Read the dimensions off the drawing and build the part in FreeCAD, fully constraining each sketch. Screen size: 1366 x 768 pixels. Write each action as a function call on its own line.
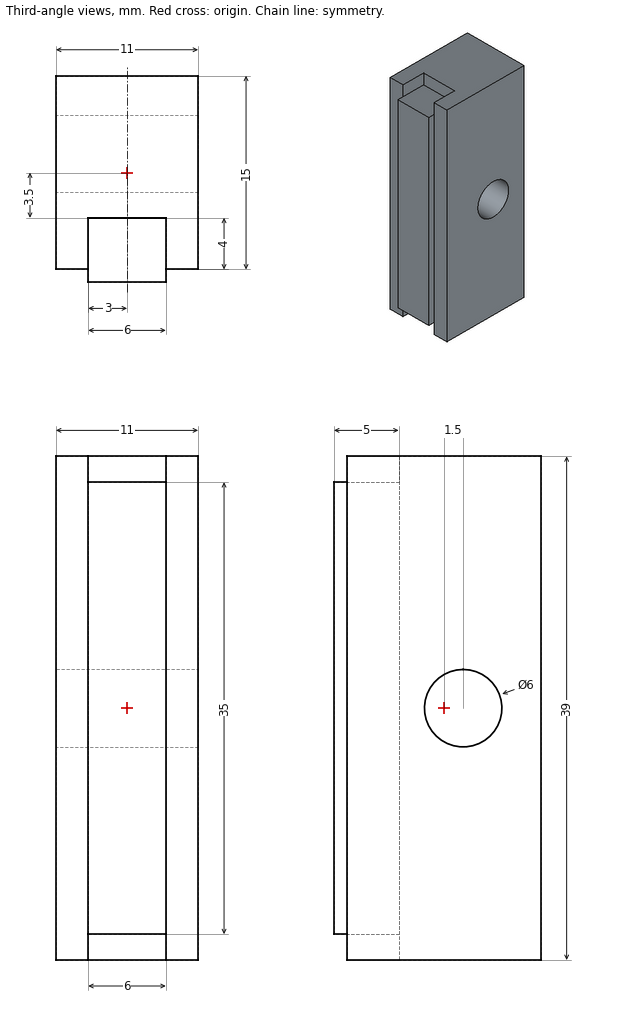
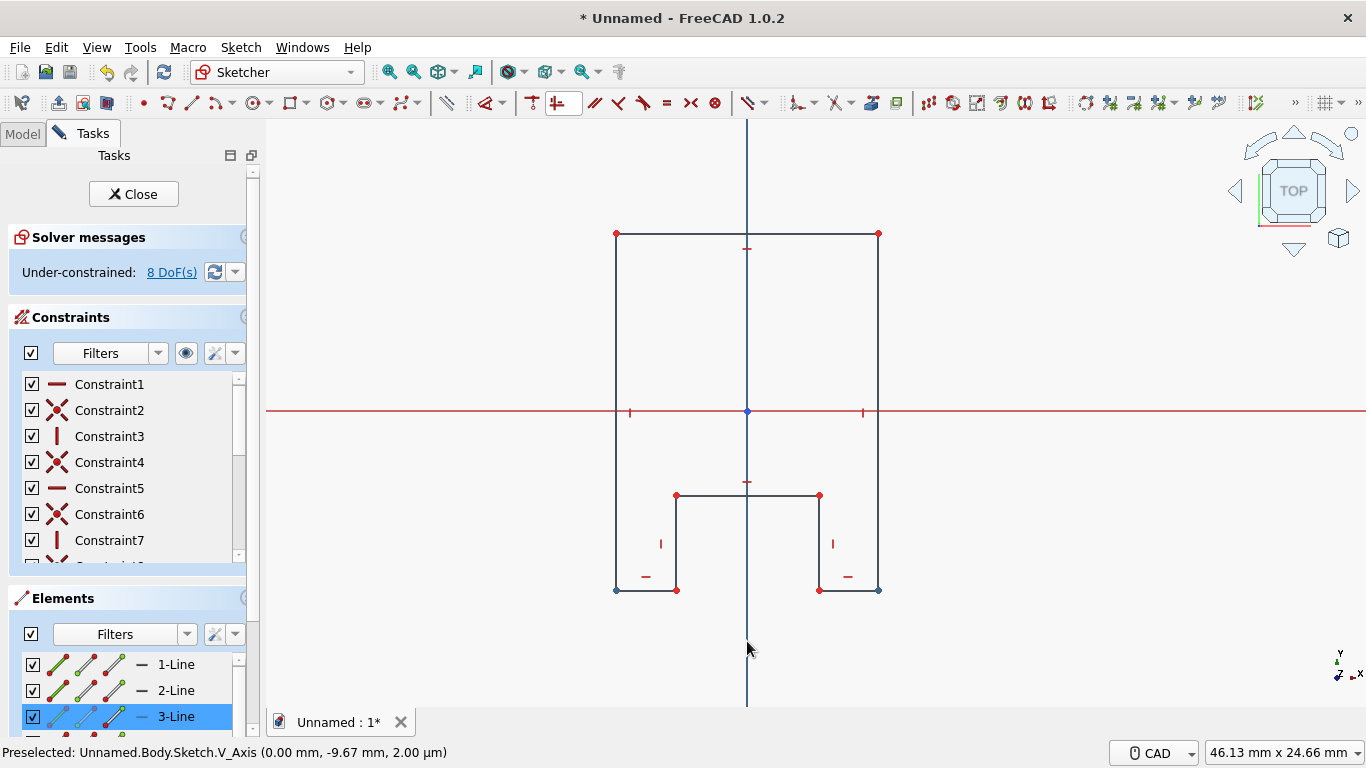
click(692, 104)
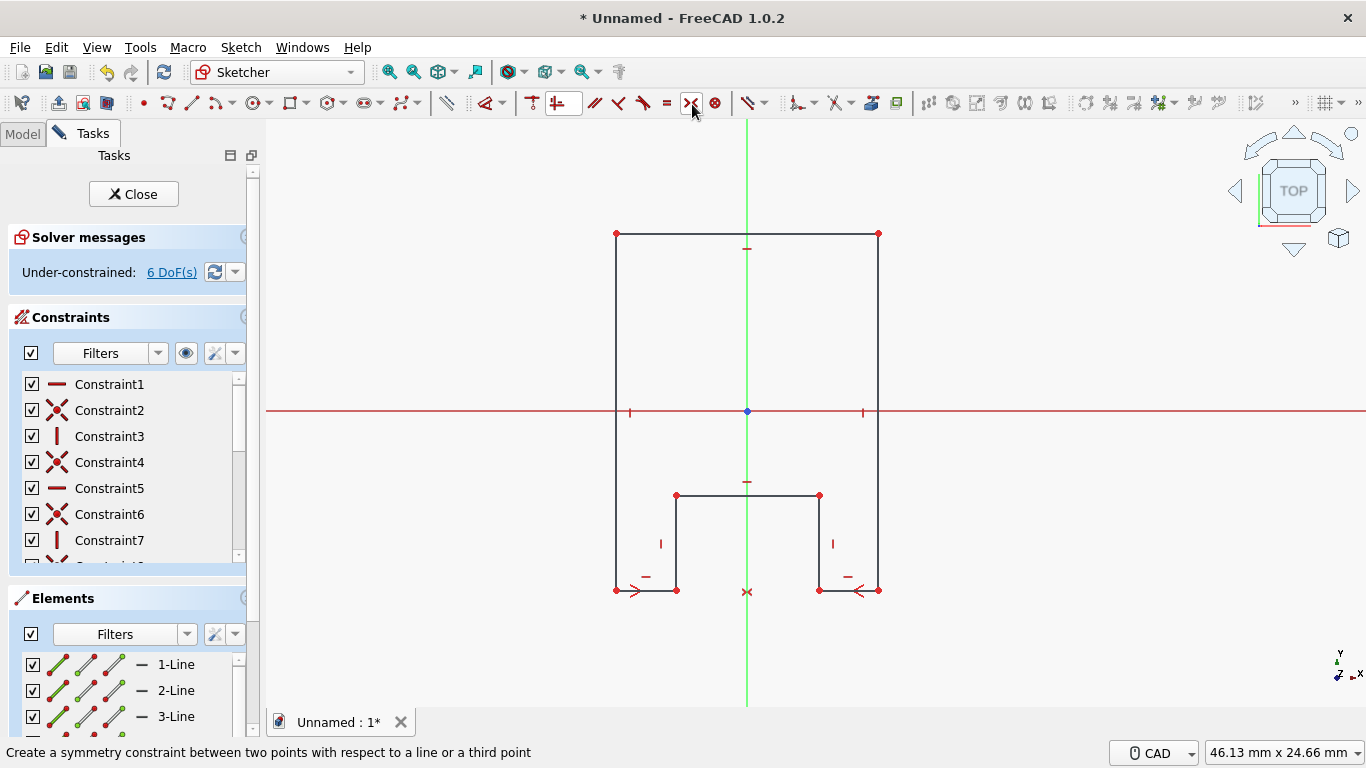
click(486, 104)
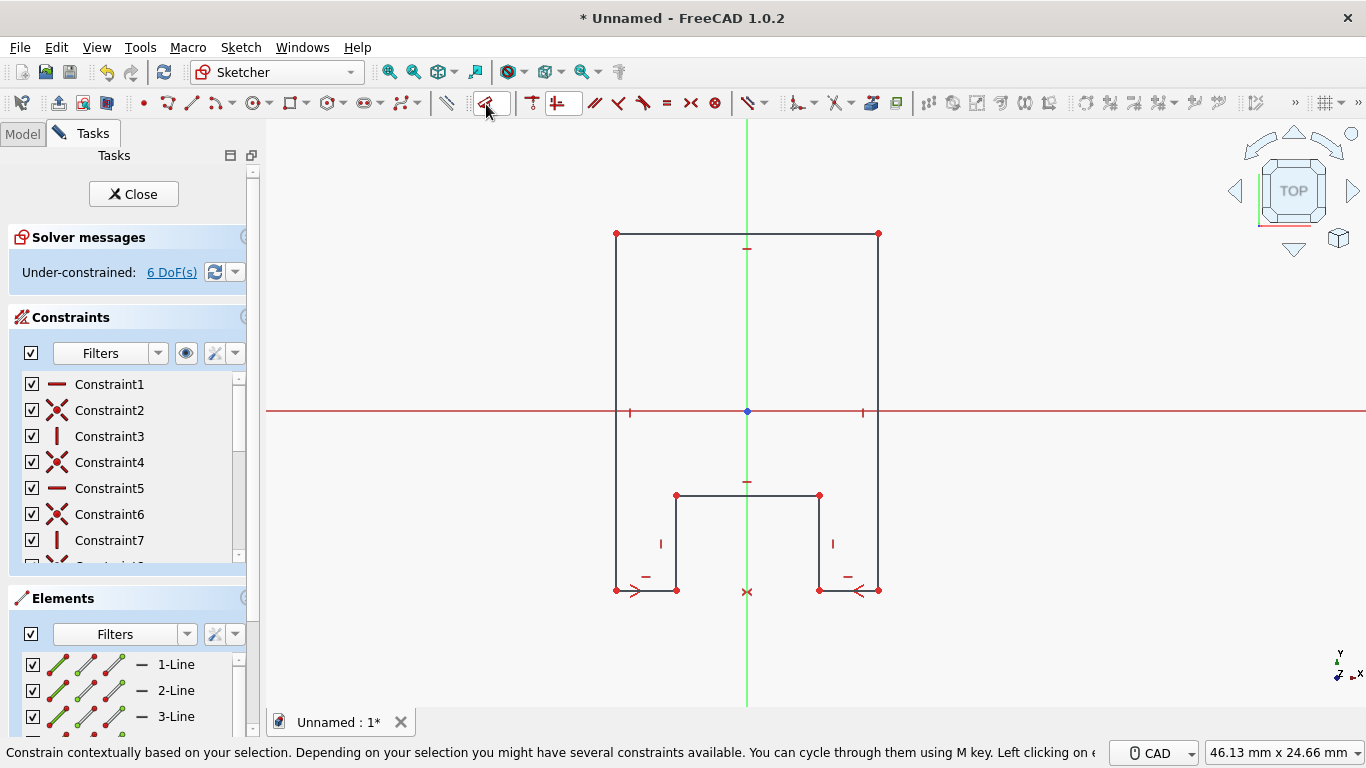
click(719, 496)
click(715, 530)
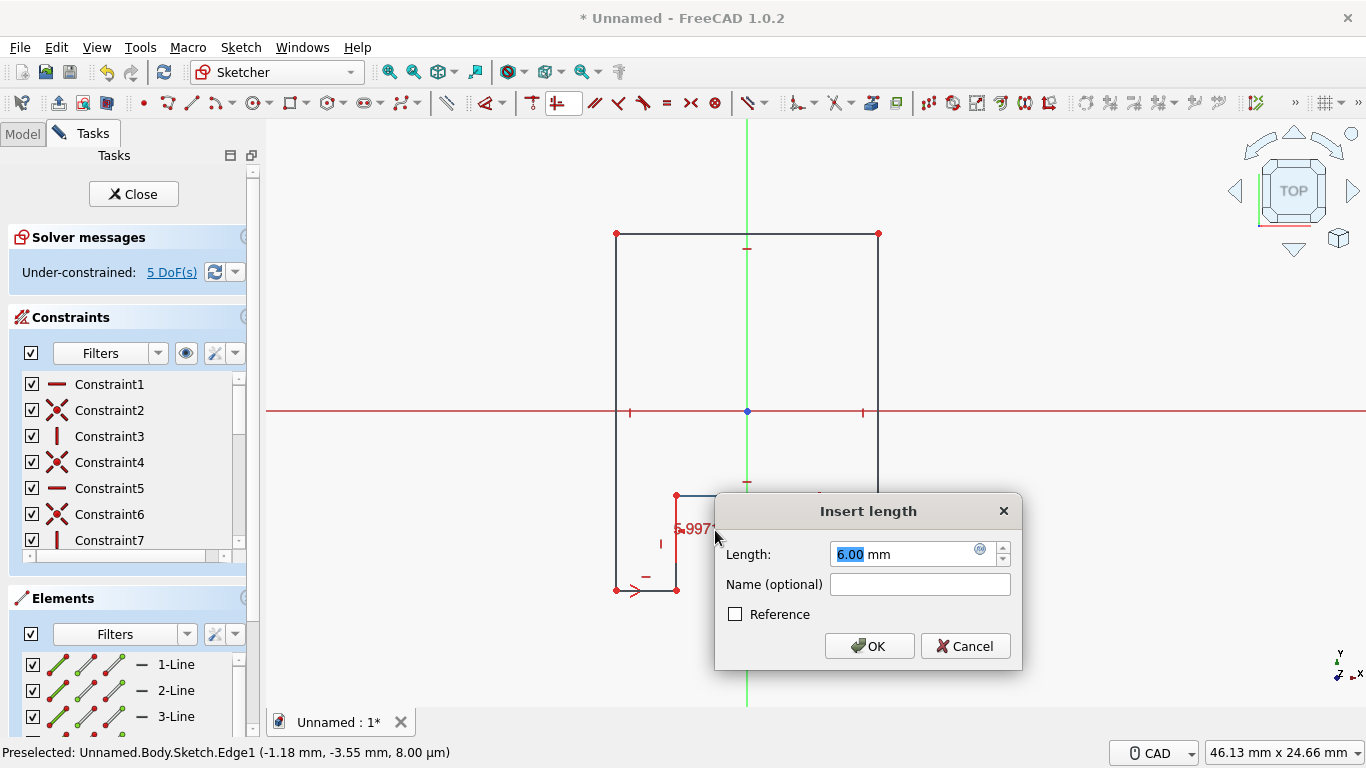
text(6)
key(Return)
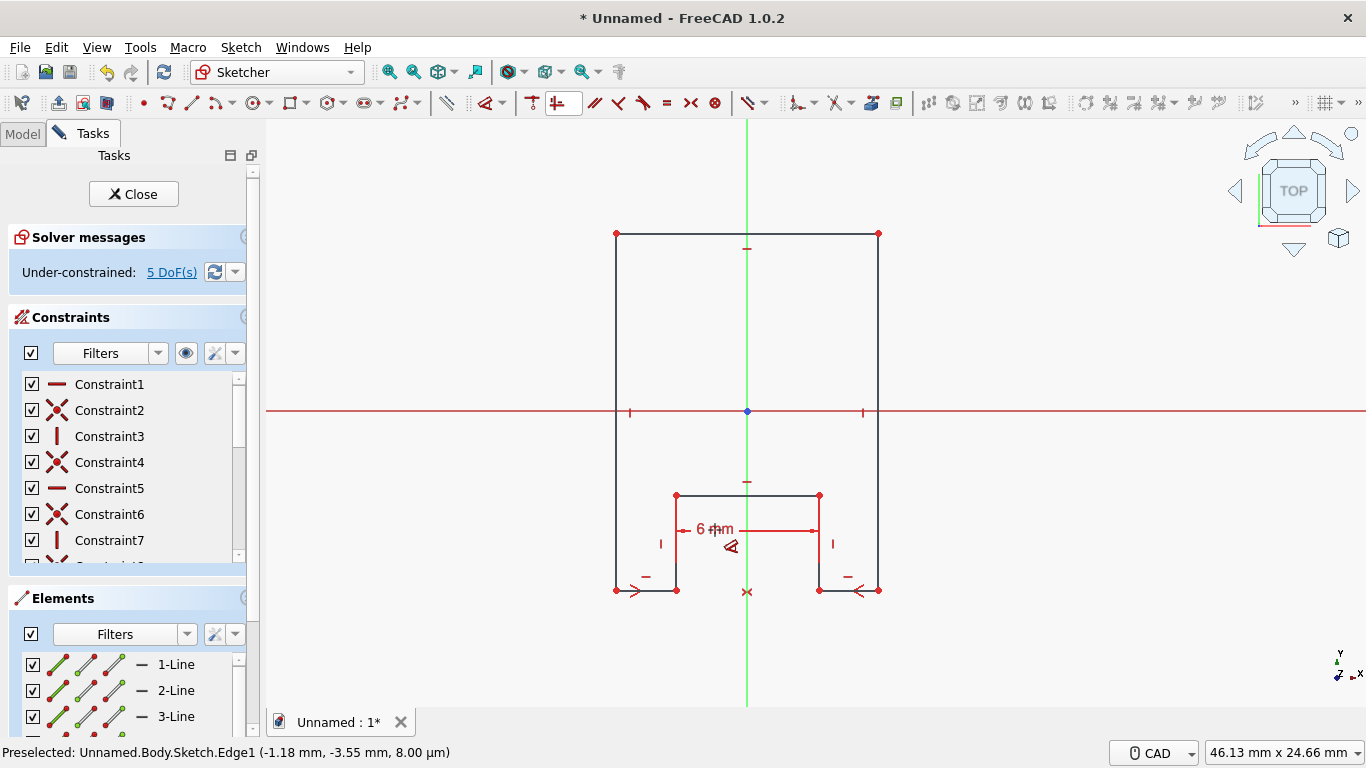
click(819, 524)
click(853, 543)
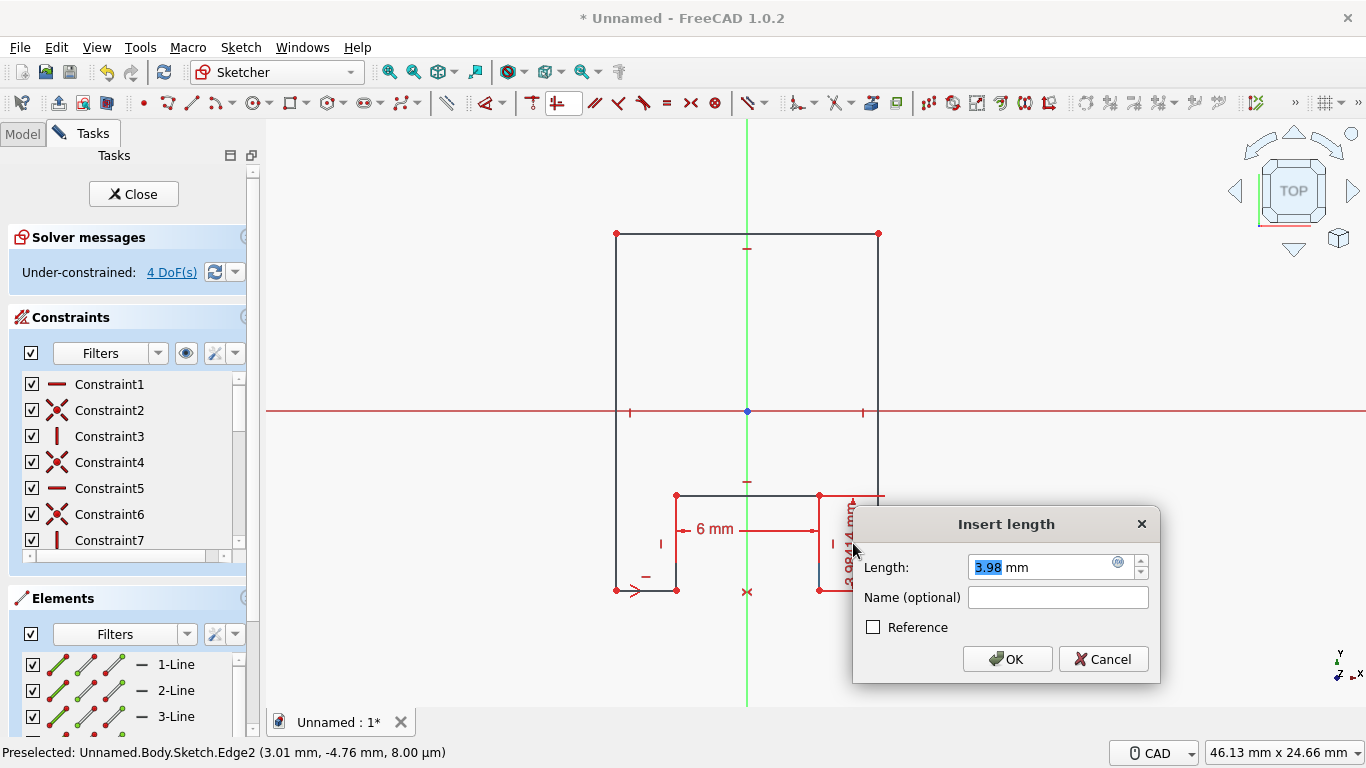
text(4)
key(Return)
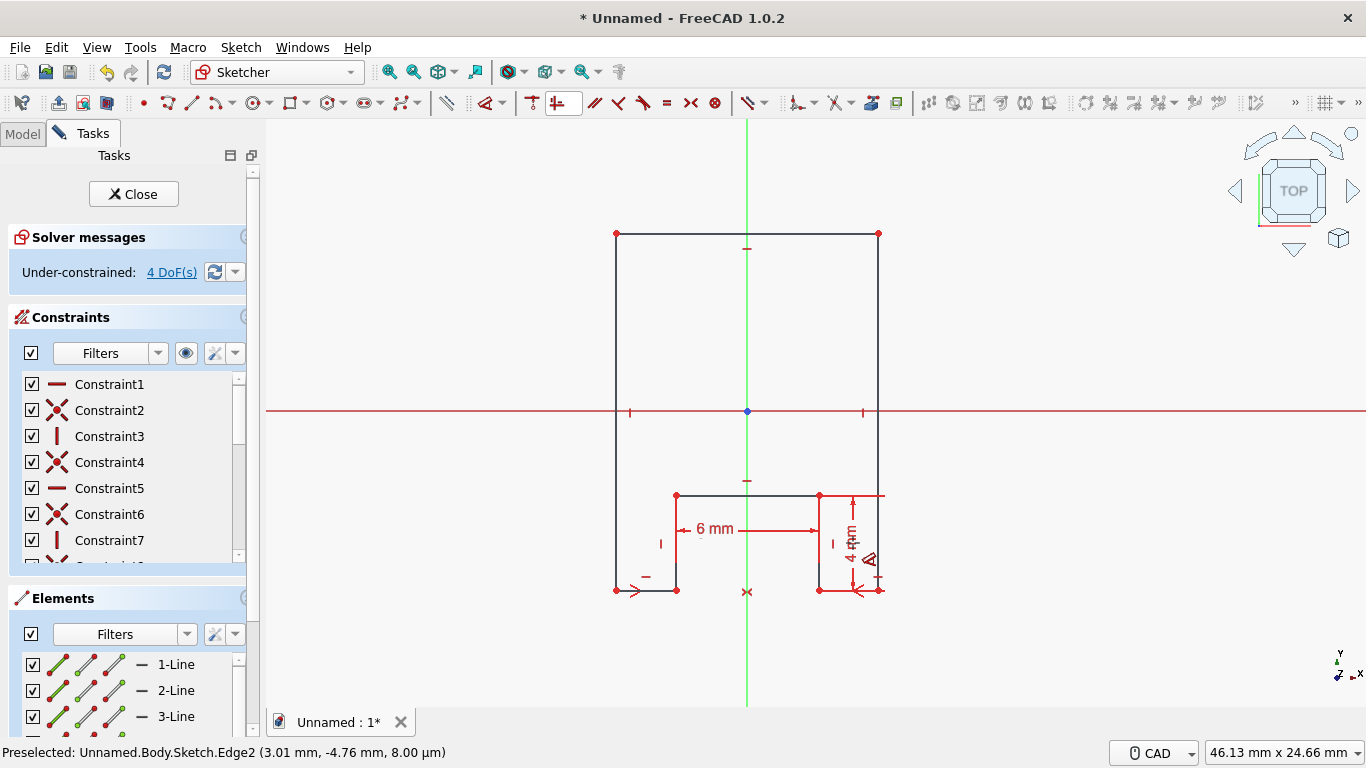
click(878, 484)
click(912, 330)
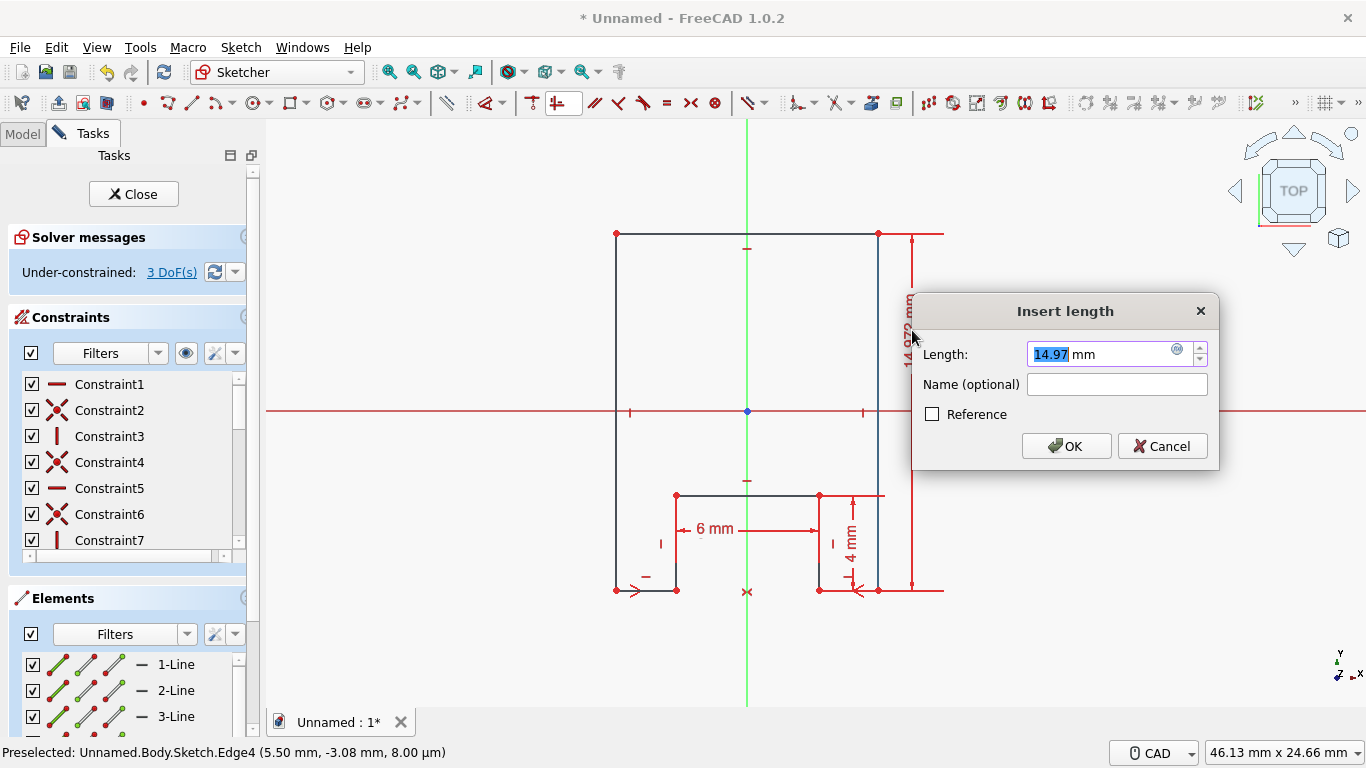
text(15)
key(Return)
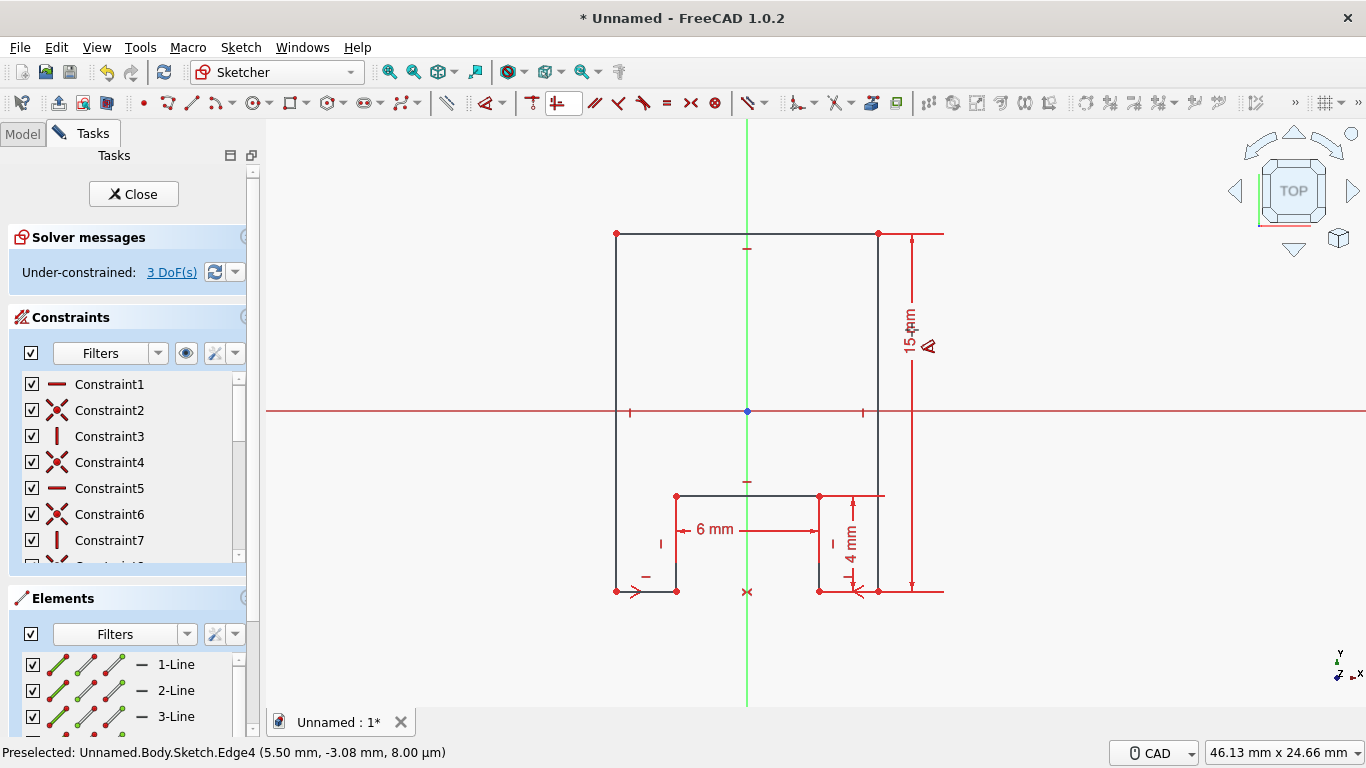
click(800, 234)
click(687, 200)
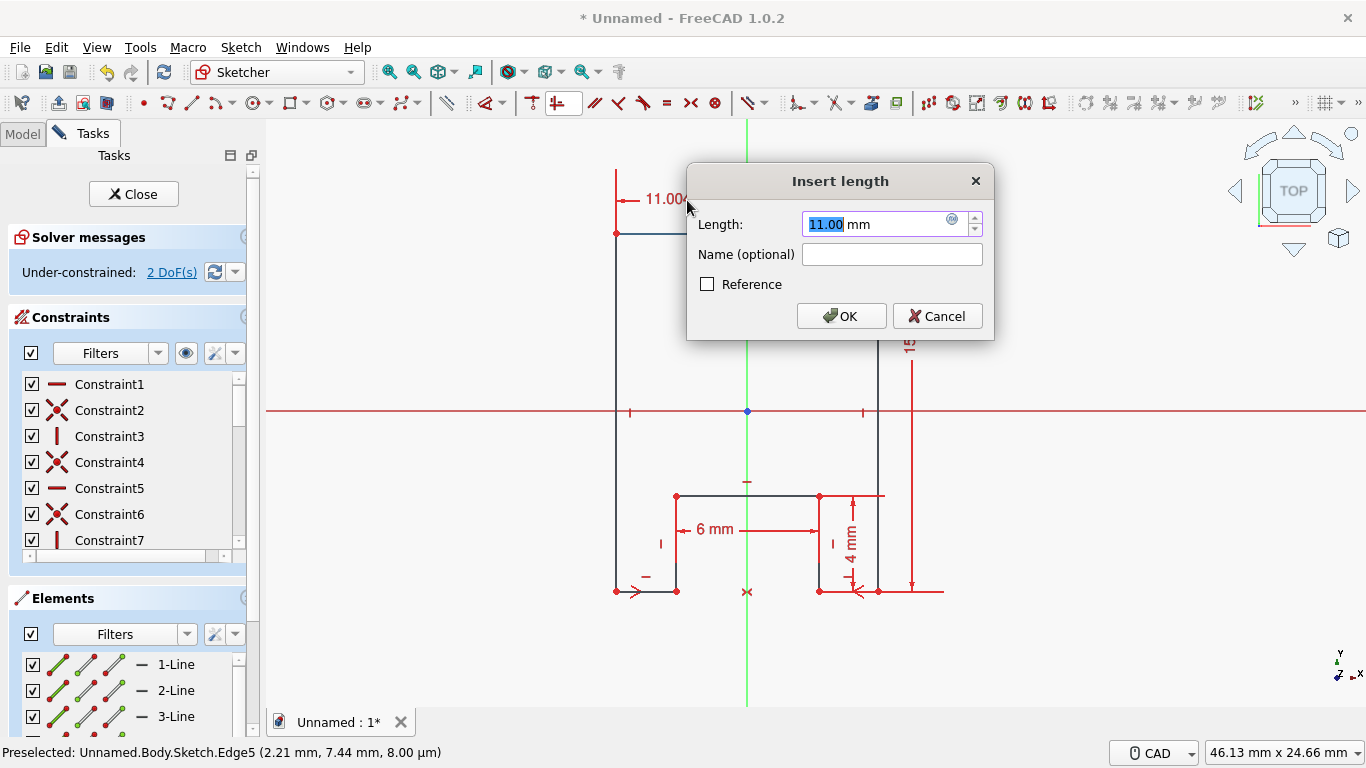
text(11)
key(Return)